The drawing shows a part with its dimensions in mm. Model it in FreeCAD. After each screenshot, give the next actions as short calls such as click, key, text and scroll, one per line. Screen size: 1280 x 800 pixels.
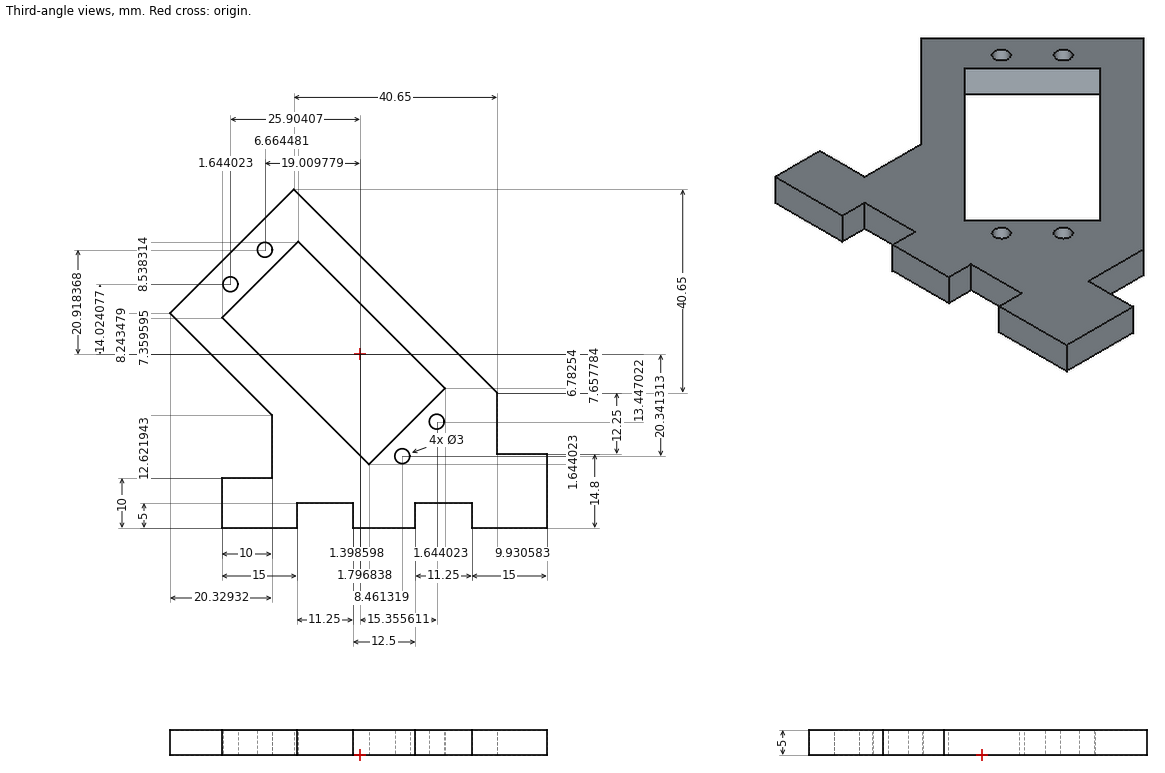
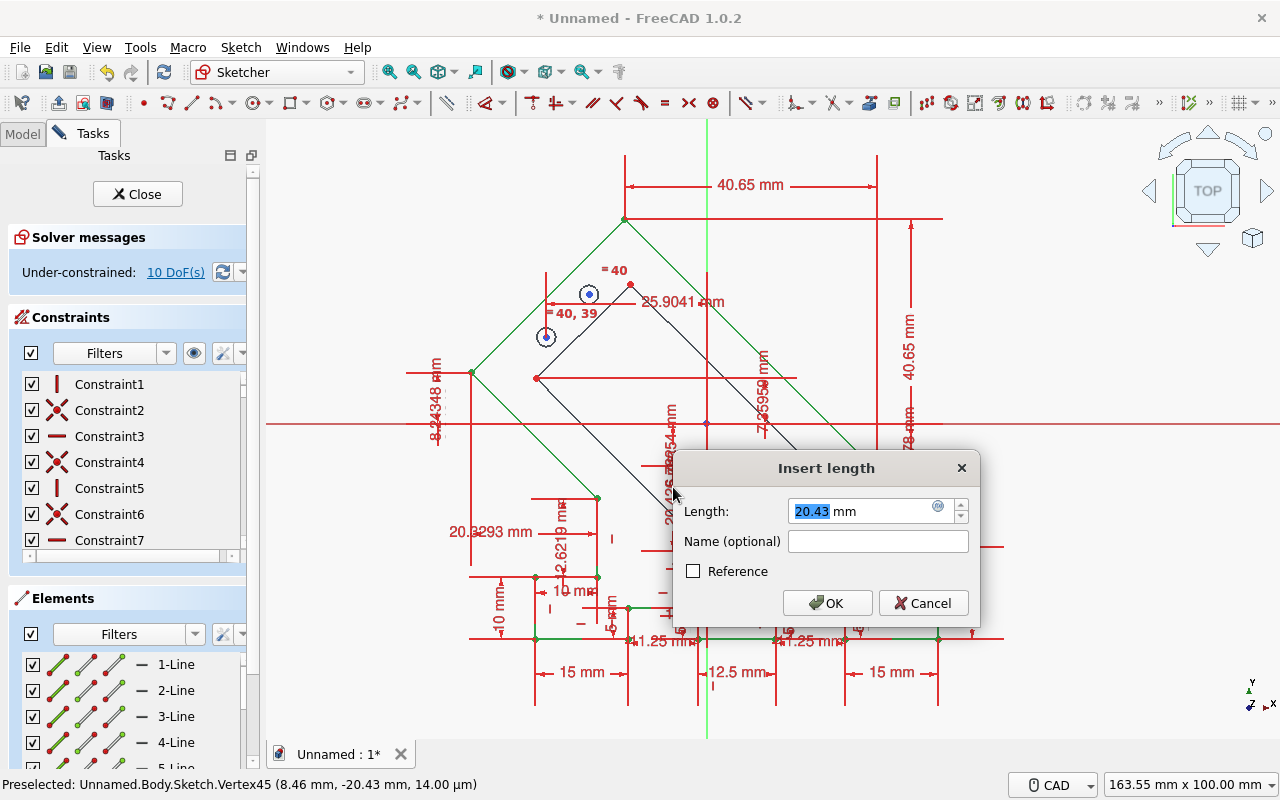
text(20.341313)
key(Return)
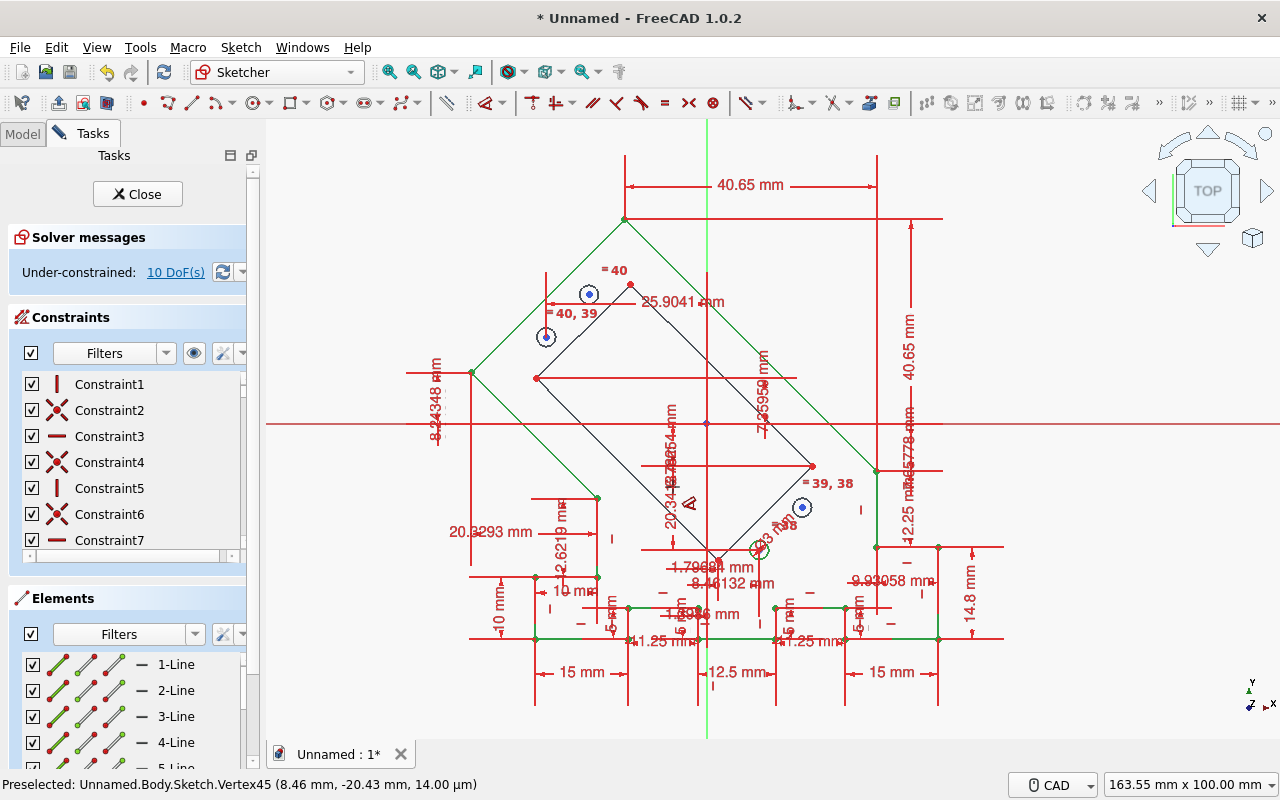
click(802, 508)
click(733, 366)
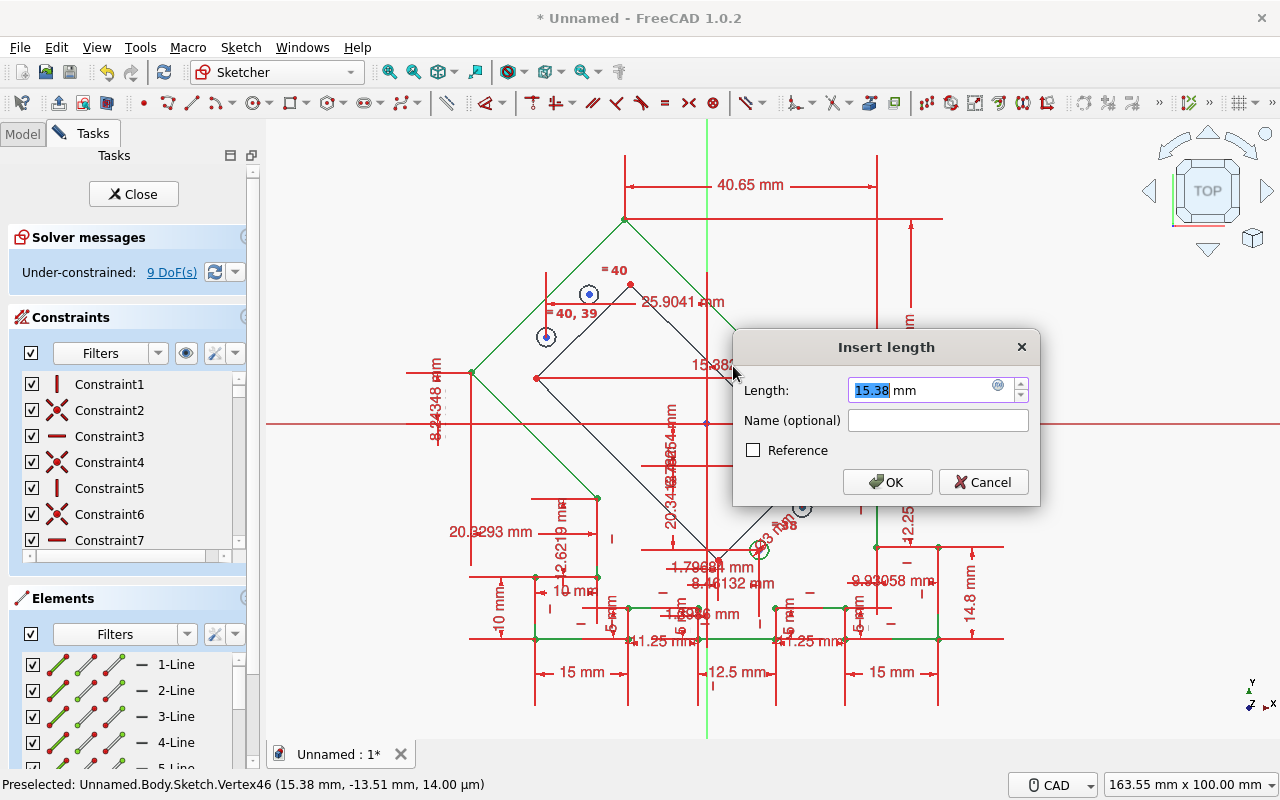
text(15.355611)
key(Return)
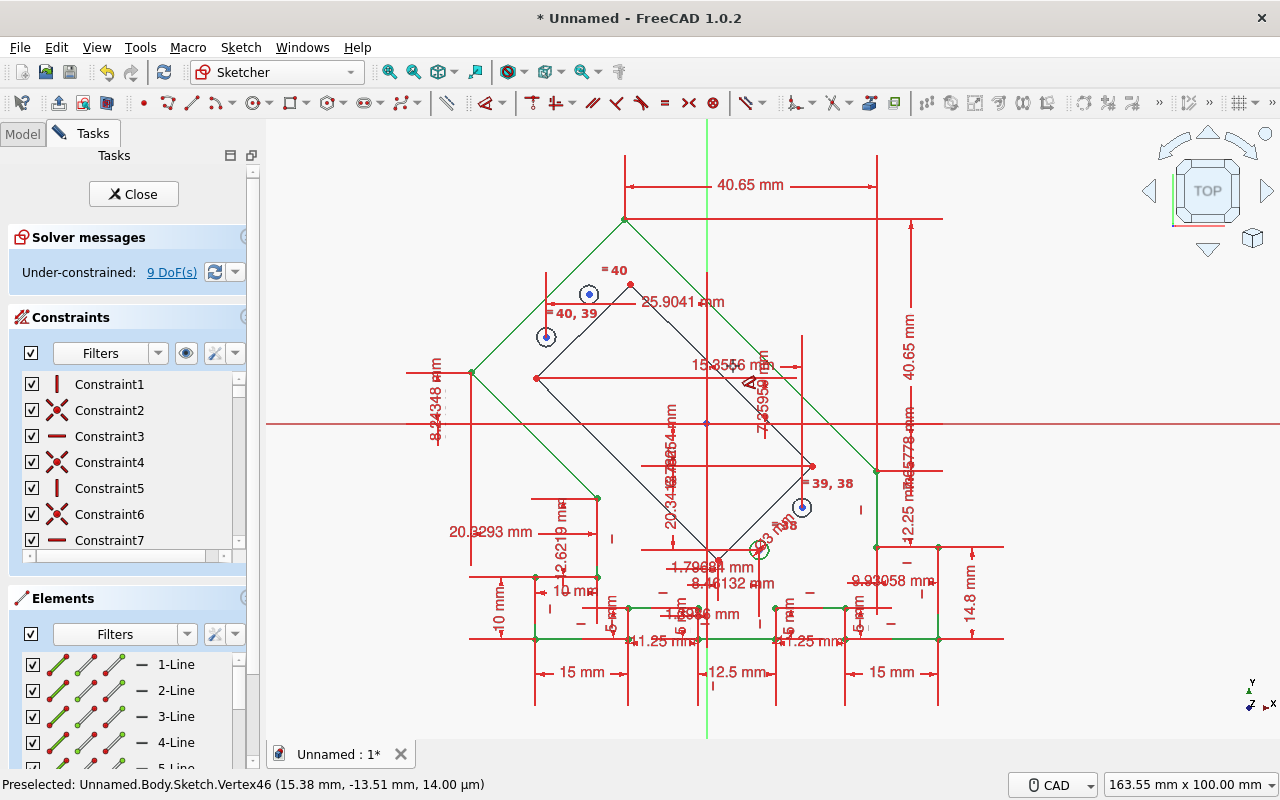
click(802, 508)
click(836, 466)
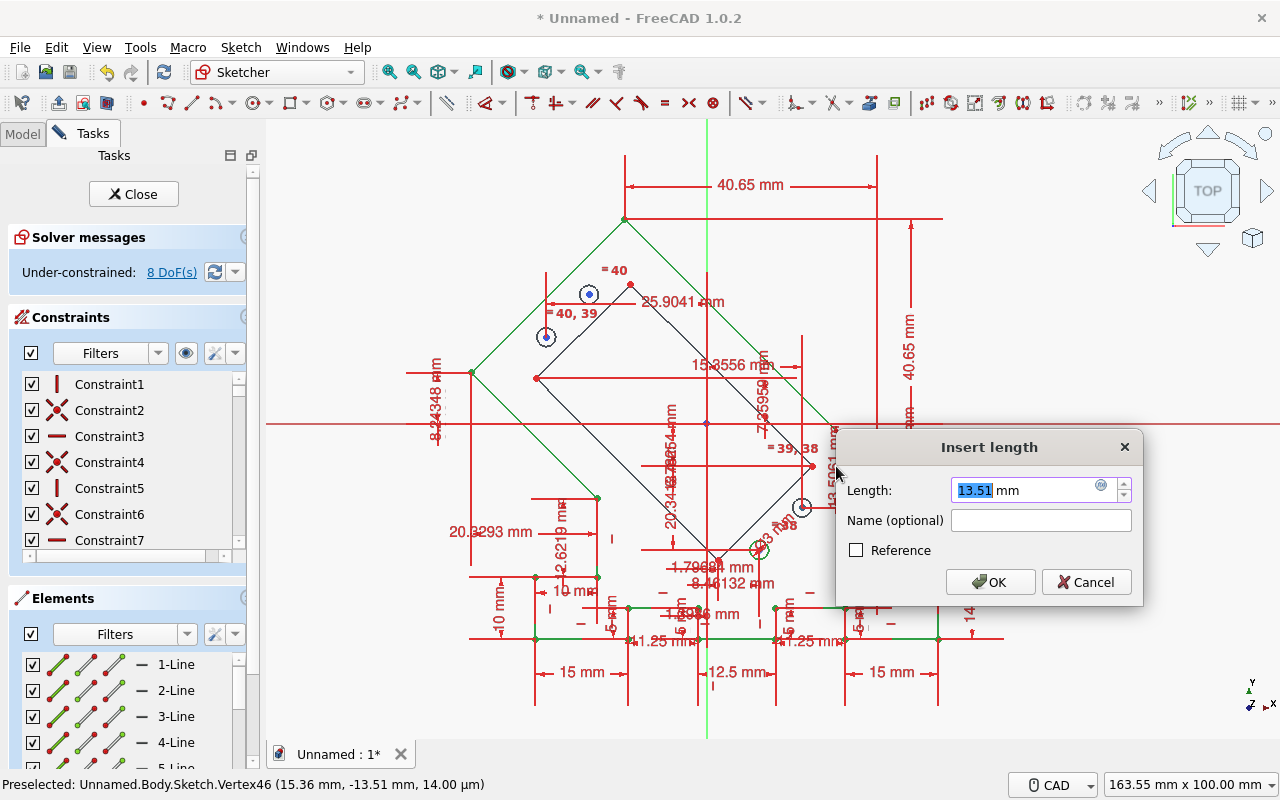
text(13.447022)
key(Return)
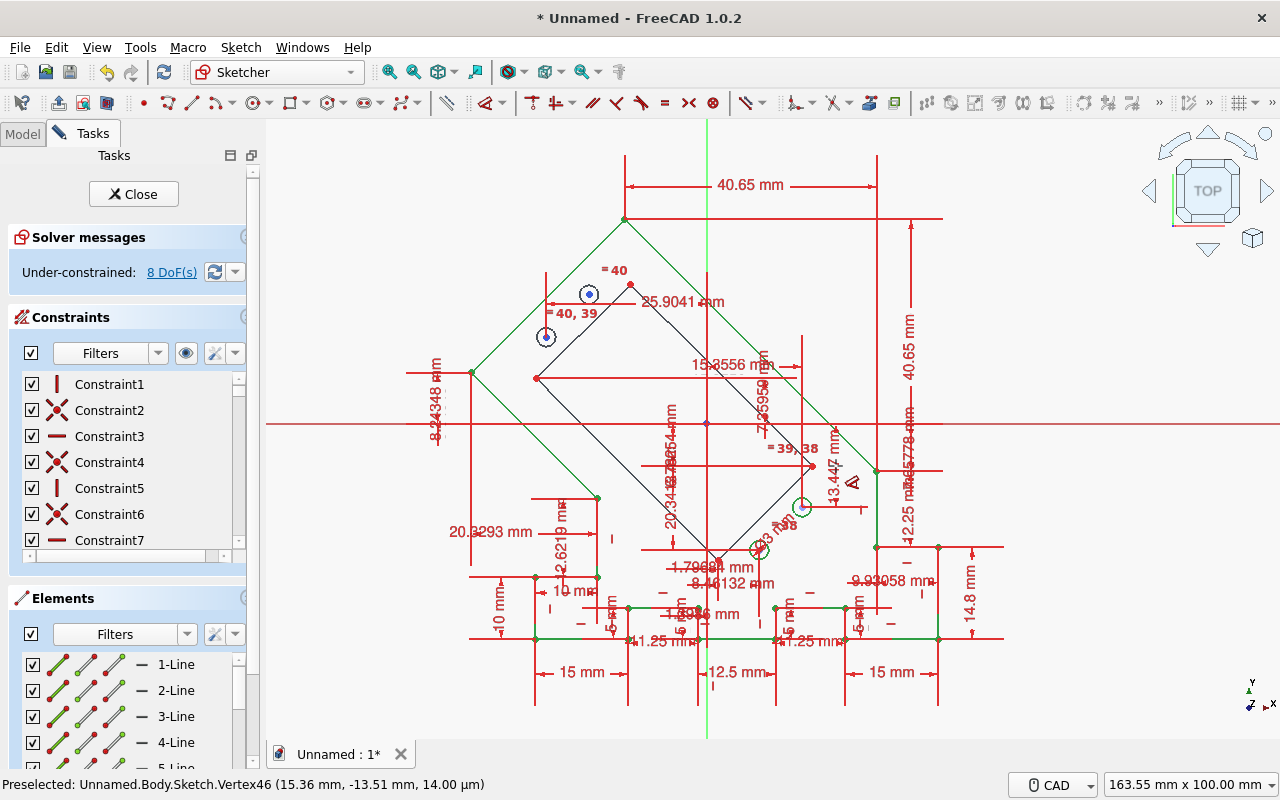
click(546, 337)
click(512, 381)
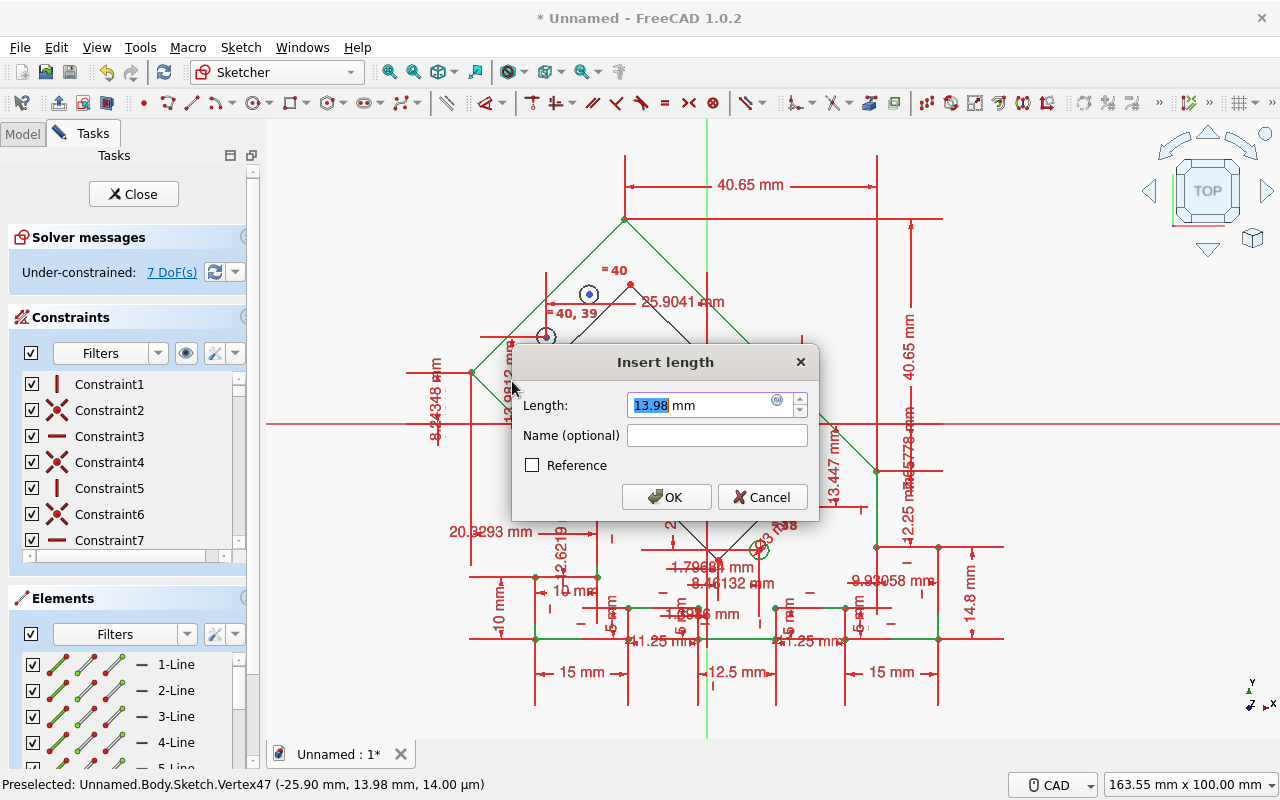
text(14.024077)
key(Return)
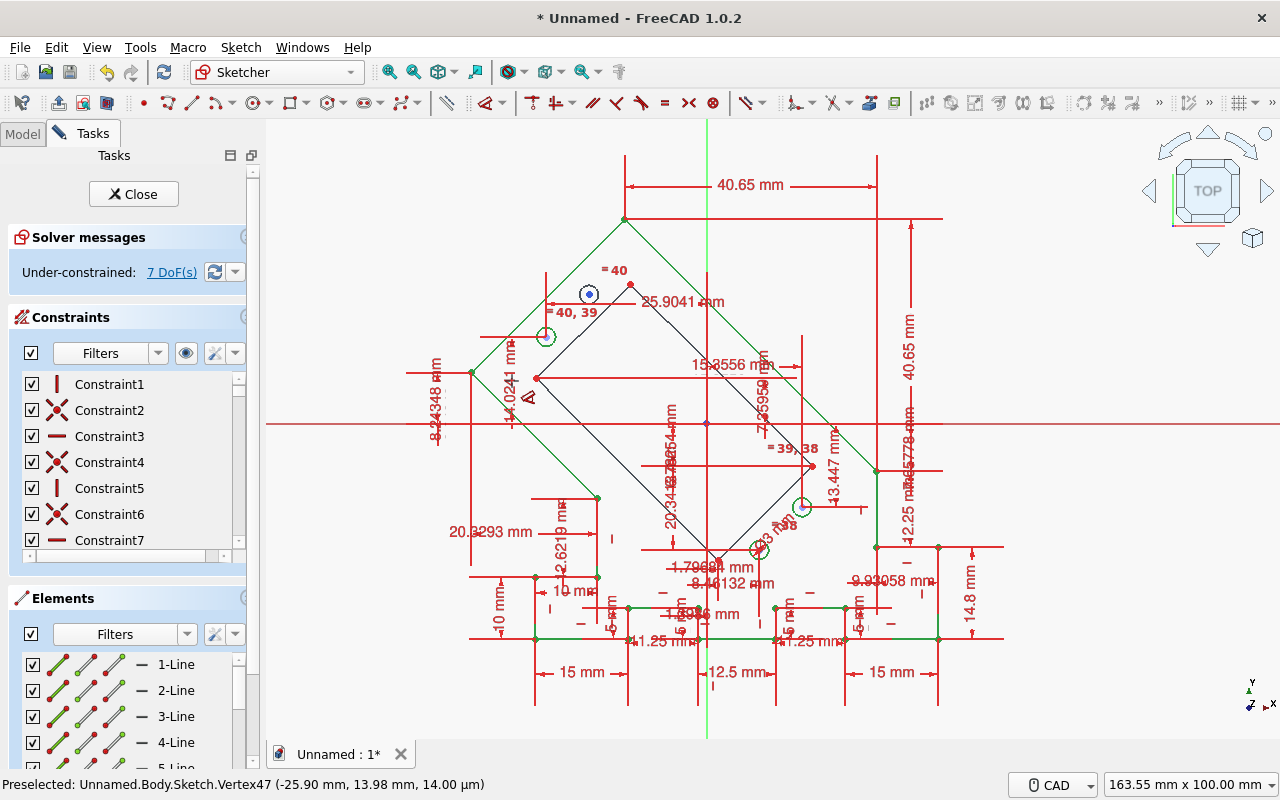
click(589, 295)
click(621, 261)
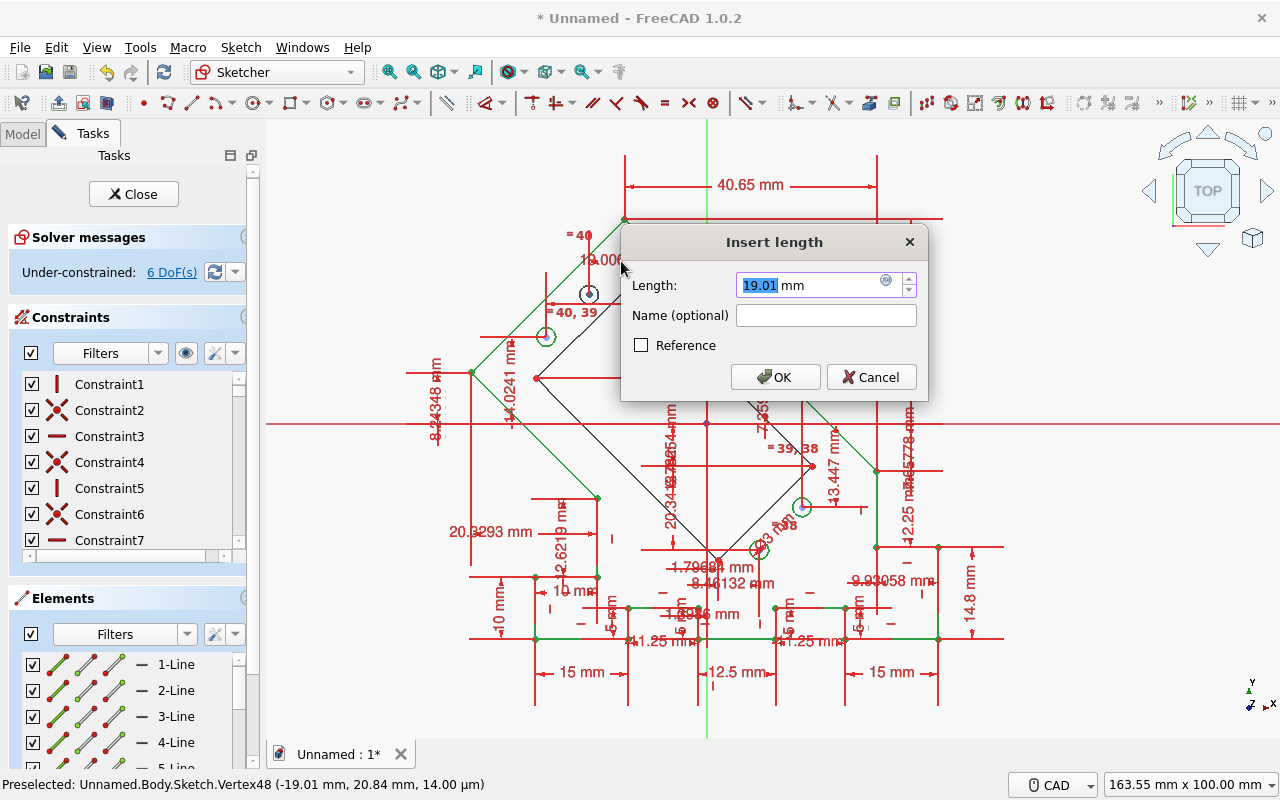
text(19.009779)
key(Return)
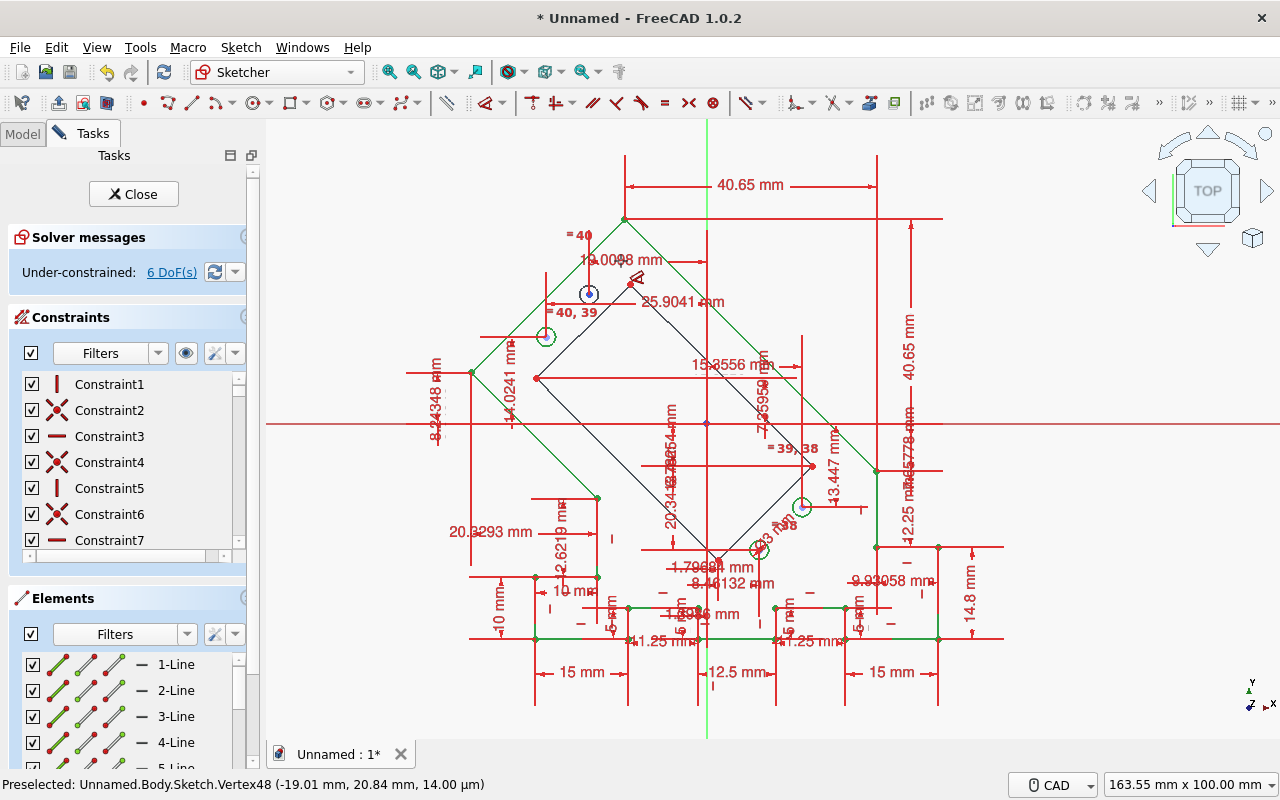
click(589, 295)
click(555, 314)